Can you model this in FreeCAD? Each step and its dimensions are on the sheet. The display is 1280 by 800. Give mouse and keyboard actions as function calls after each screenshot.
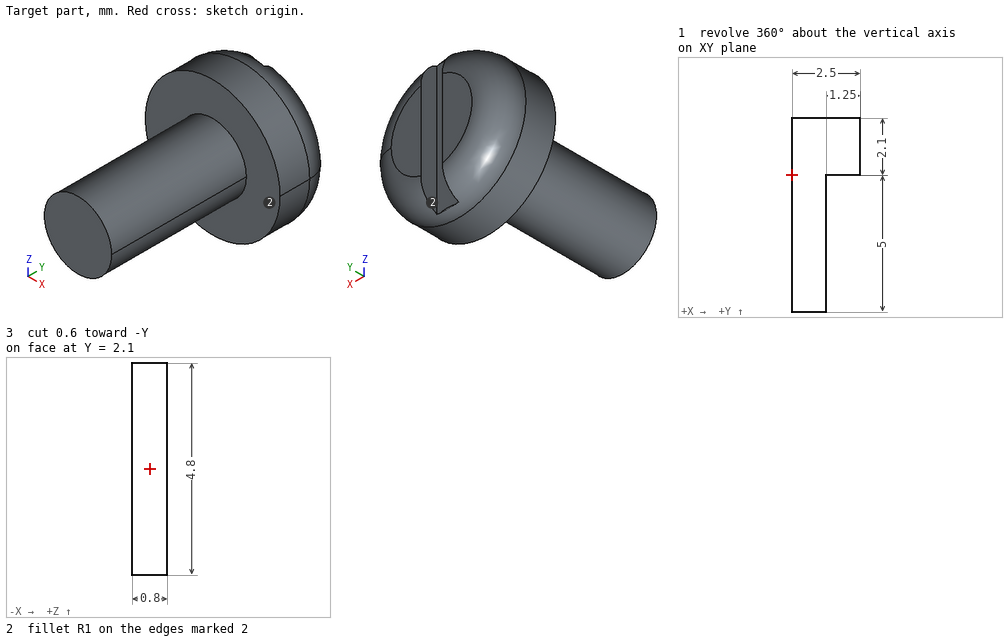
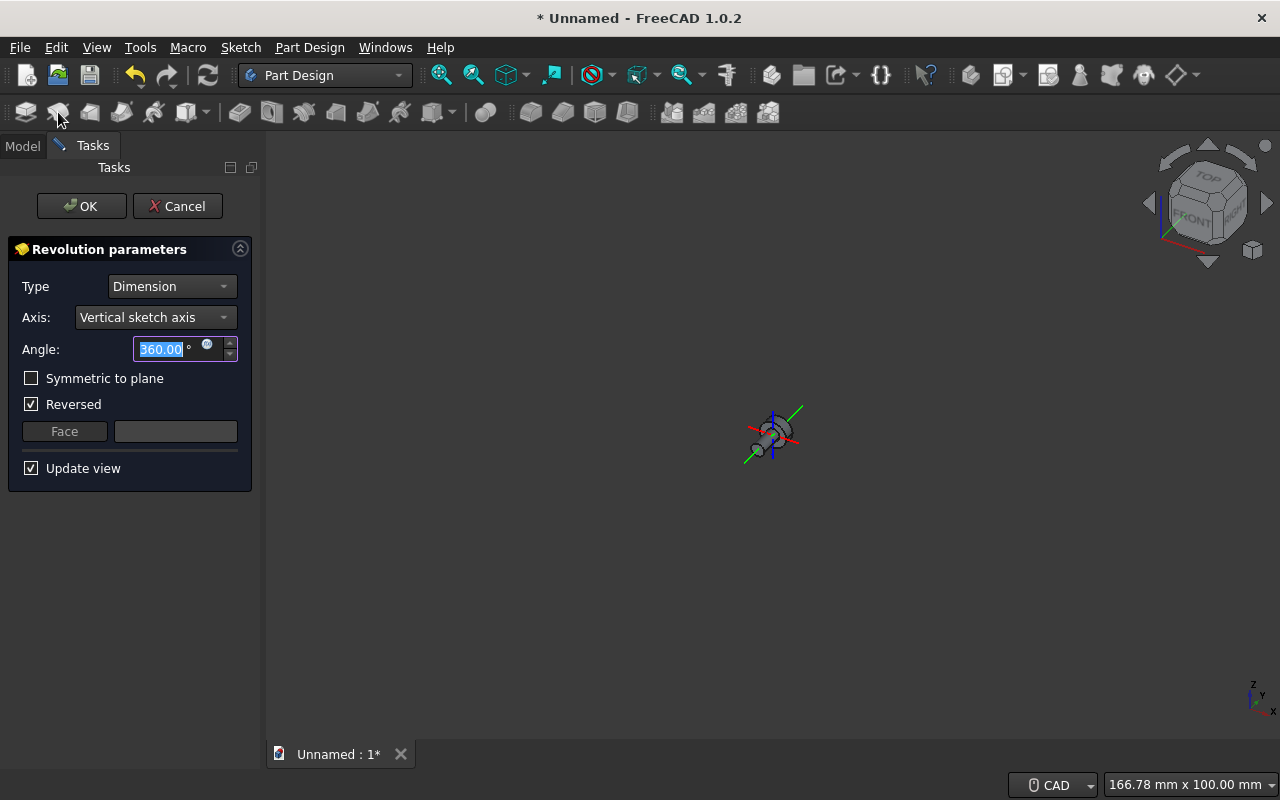
click(82, 206)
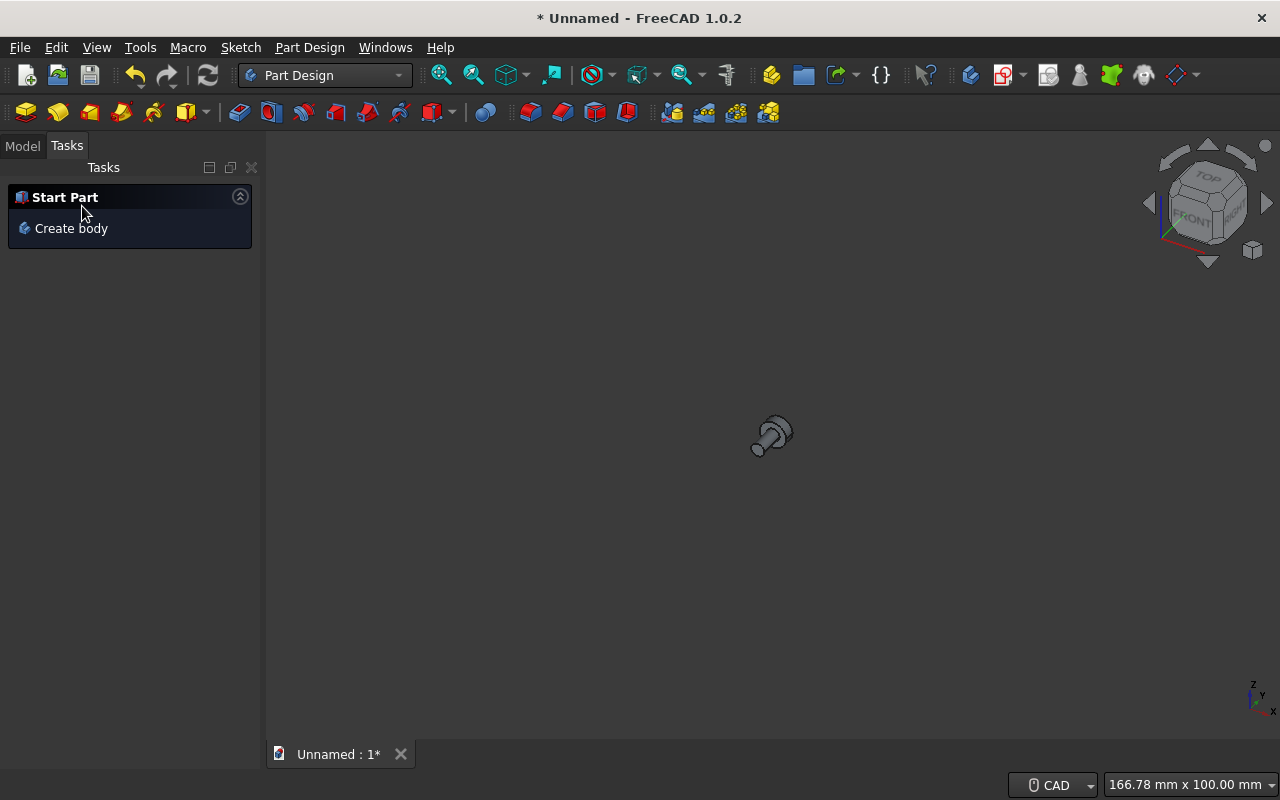
click(442, 76)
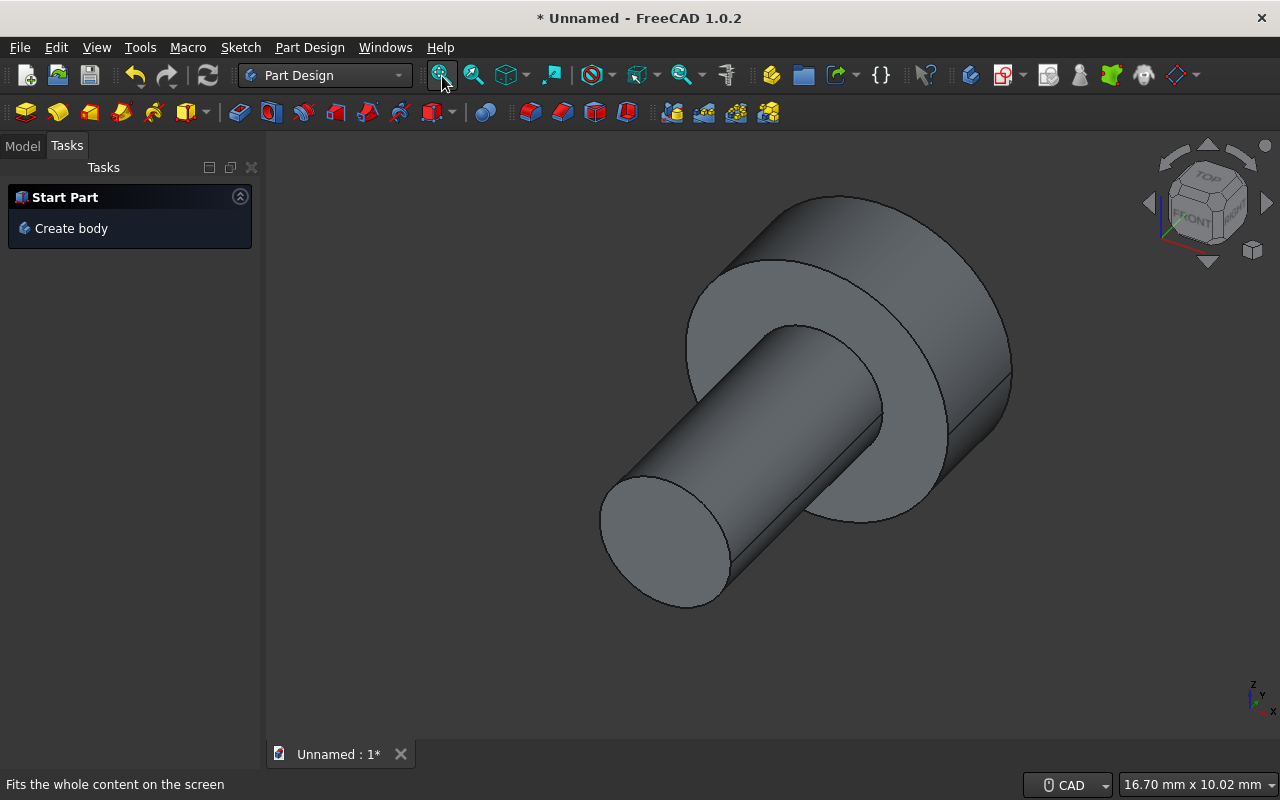
key(0)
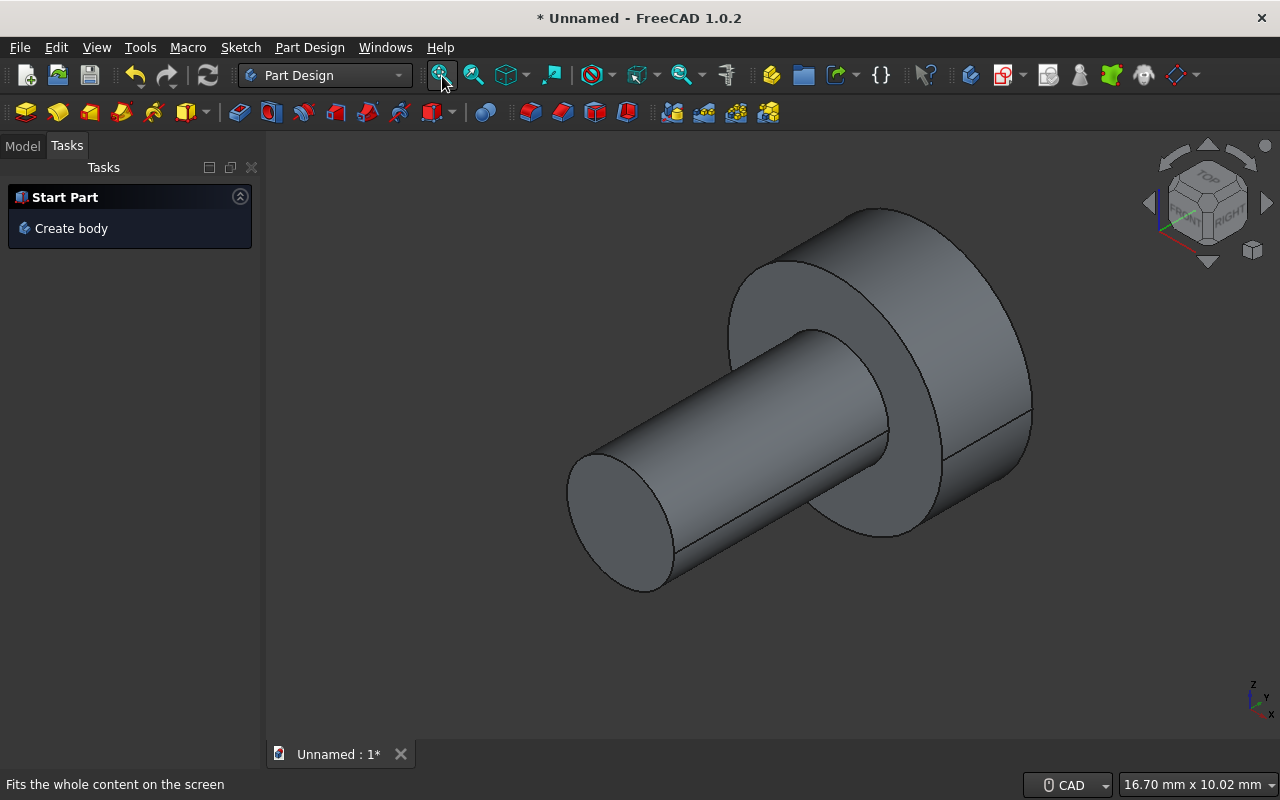
key(2)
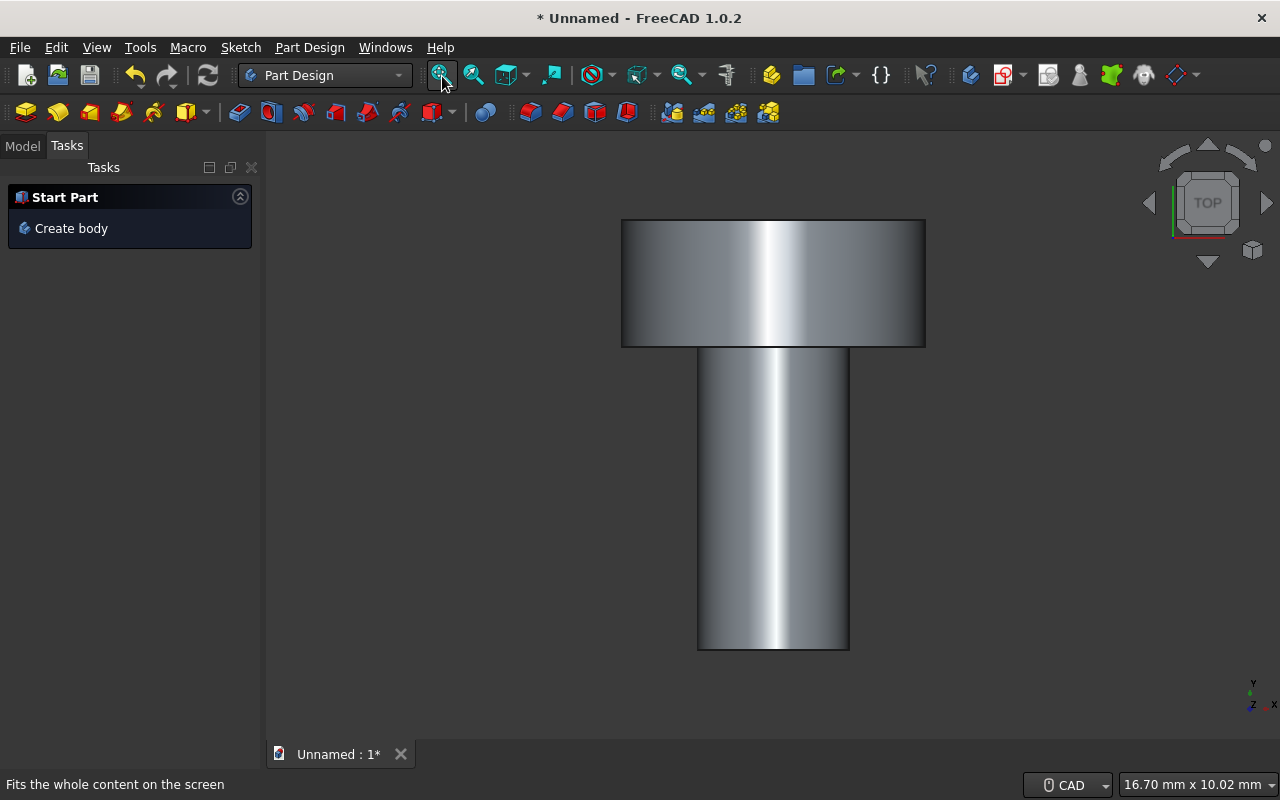
click(650, 219)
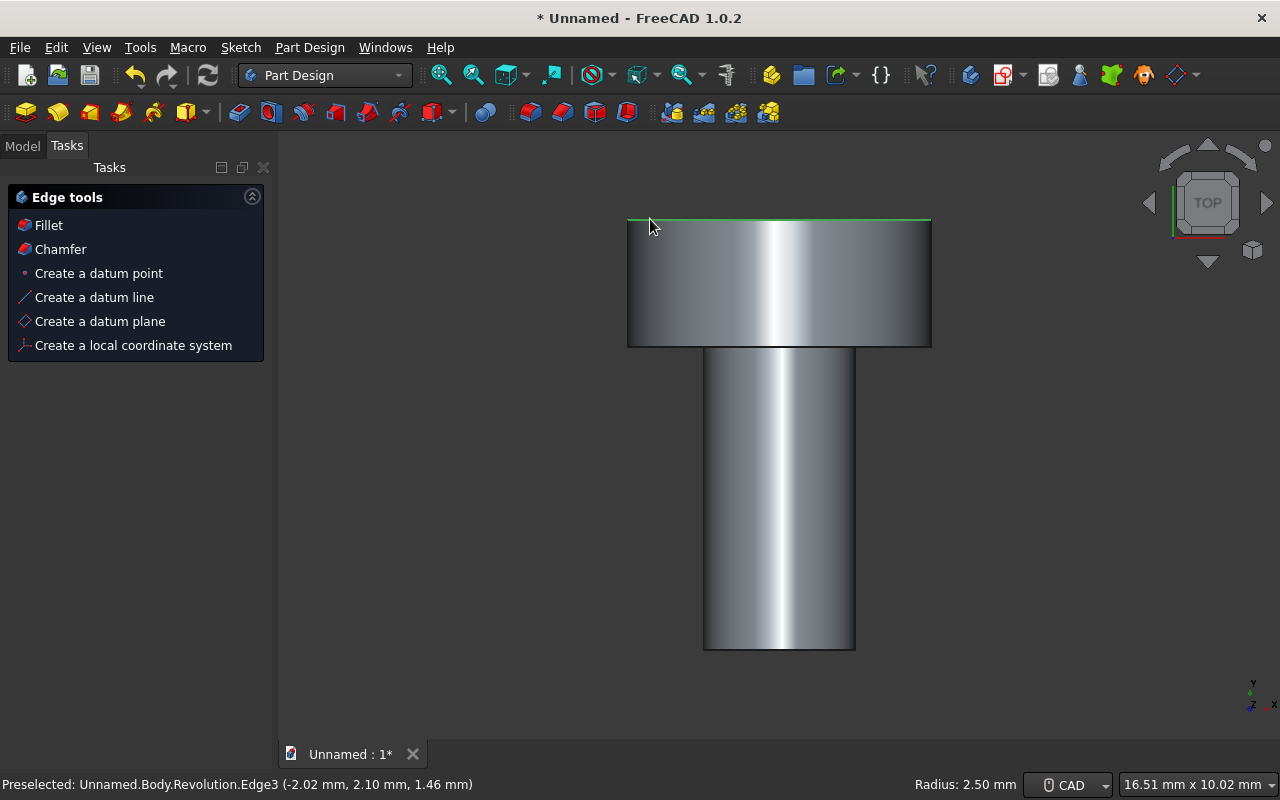
click(532, 112)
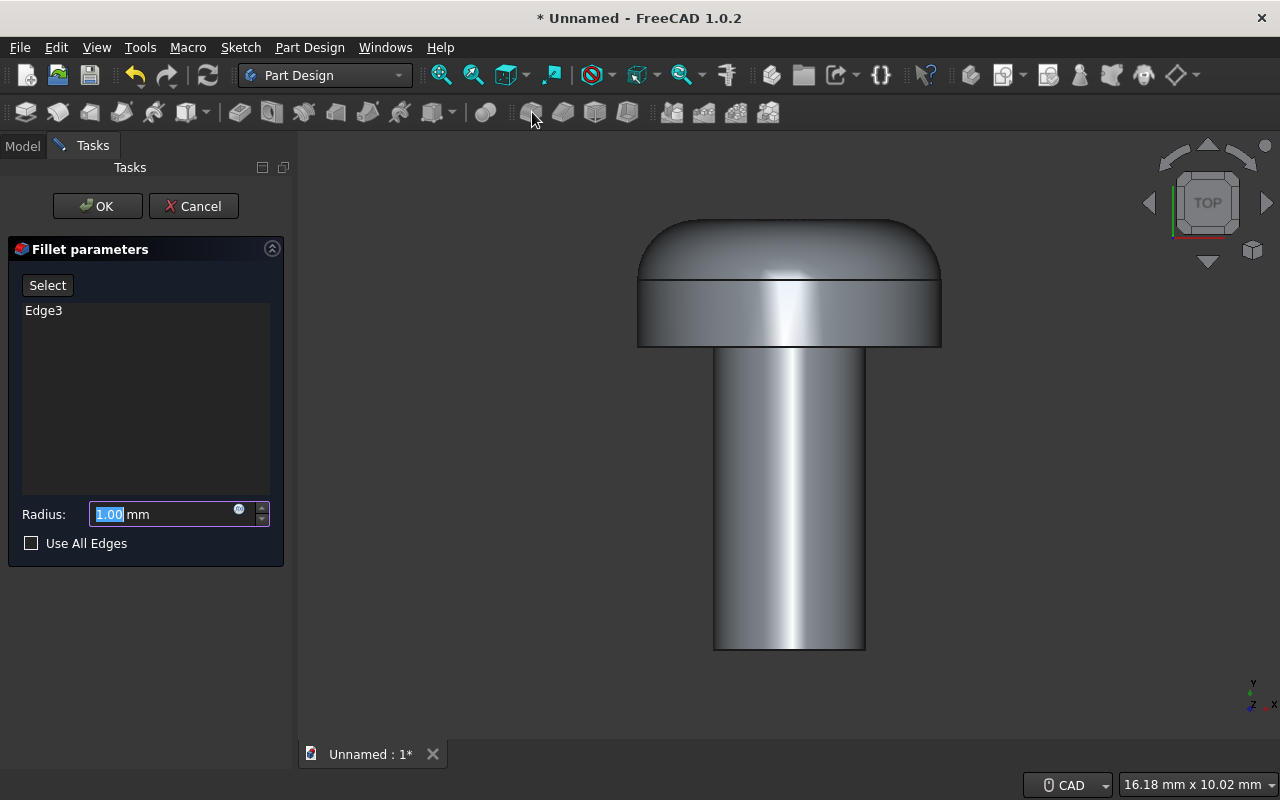
text(1)
key(Tab)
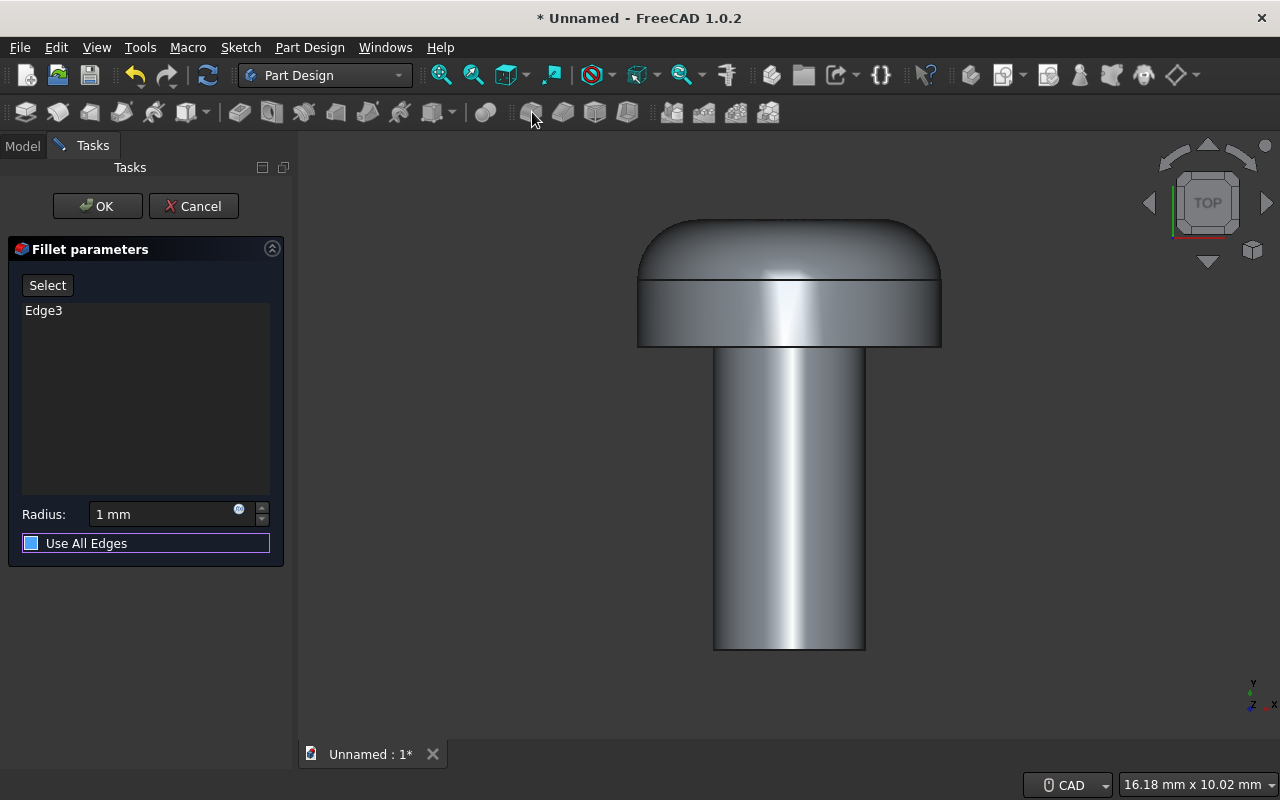
click(98, 206)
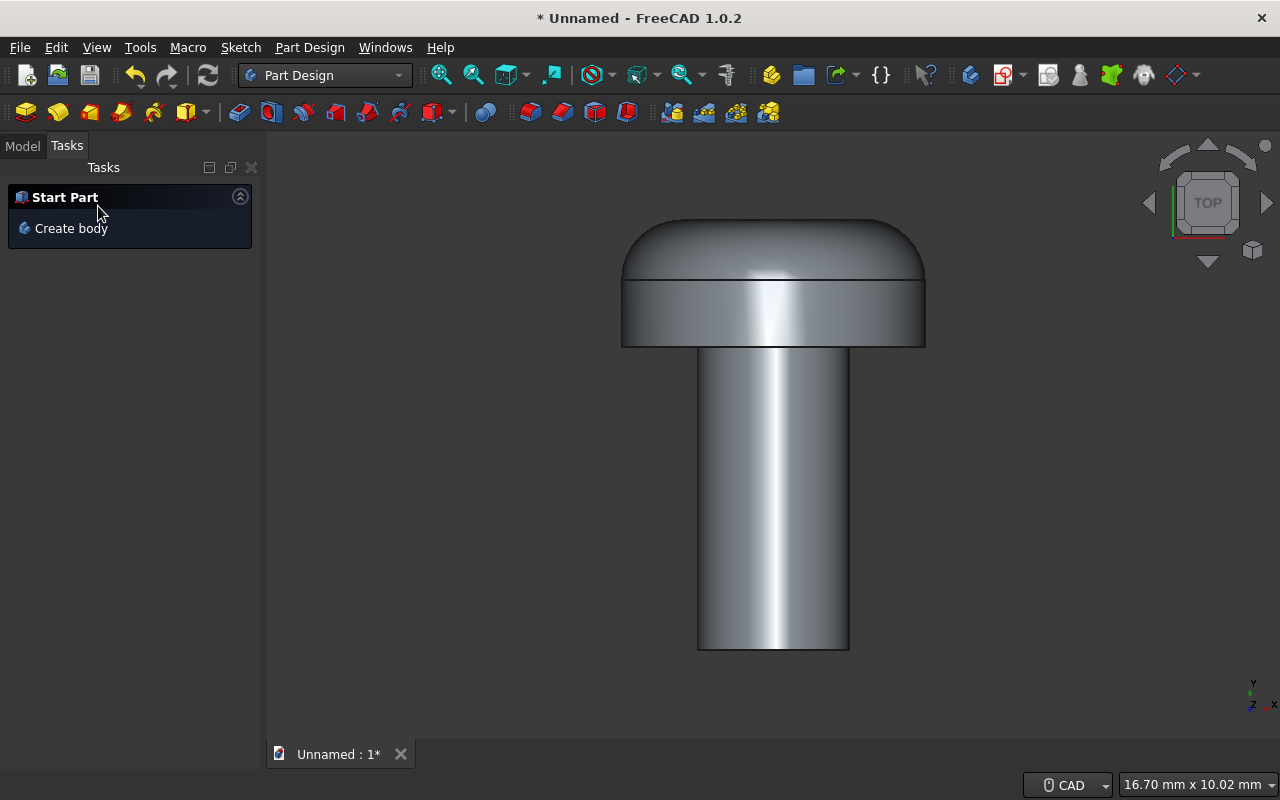
key(4)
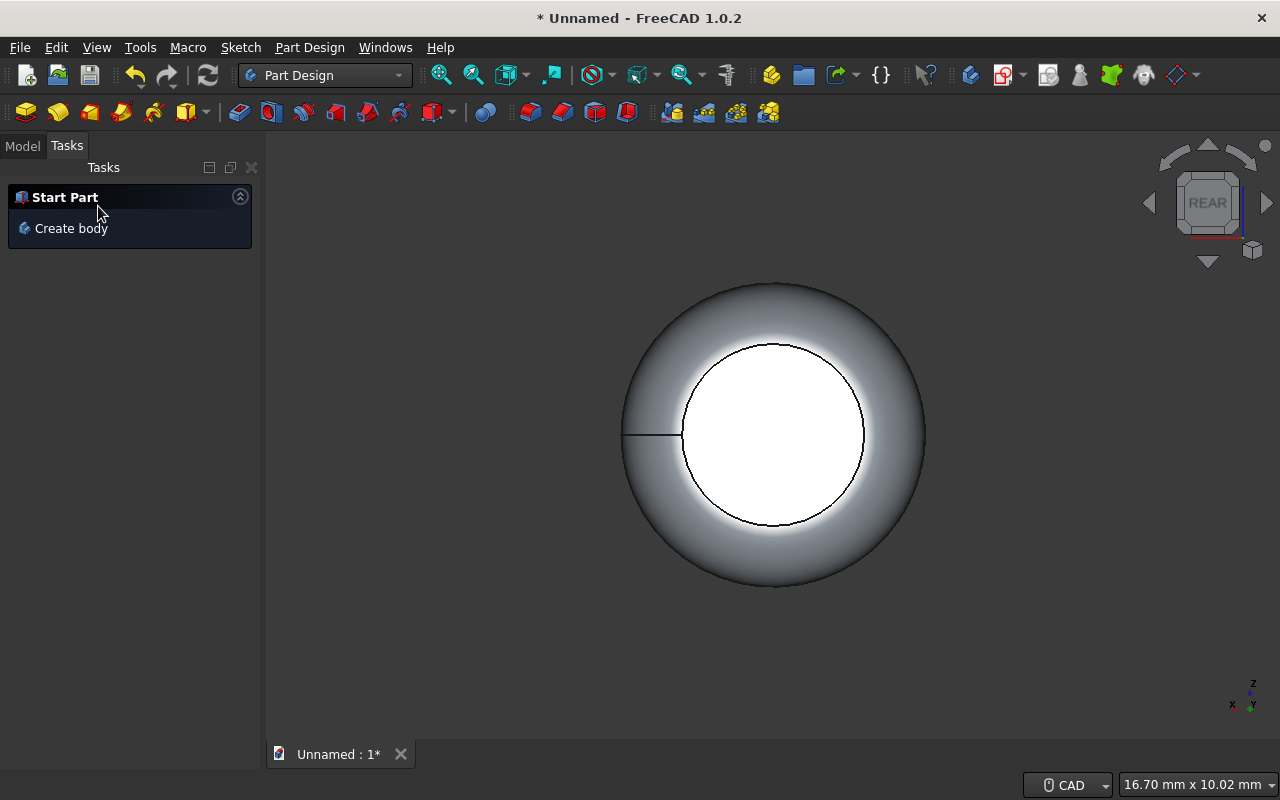
click(773, 434)